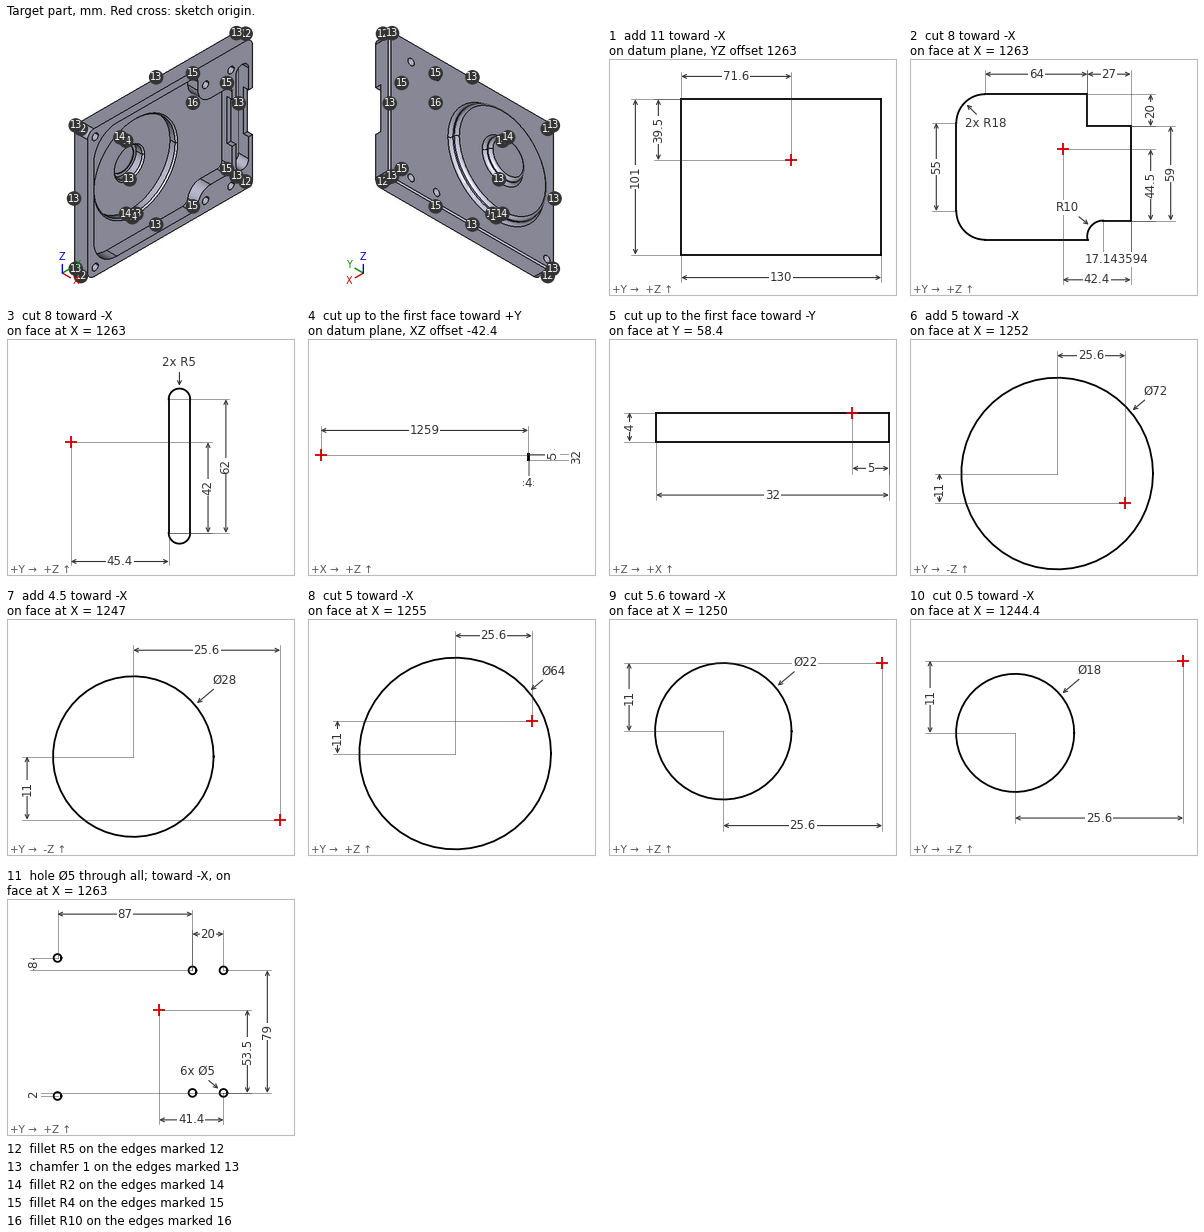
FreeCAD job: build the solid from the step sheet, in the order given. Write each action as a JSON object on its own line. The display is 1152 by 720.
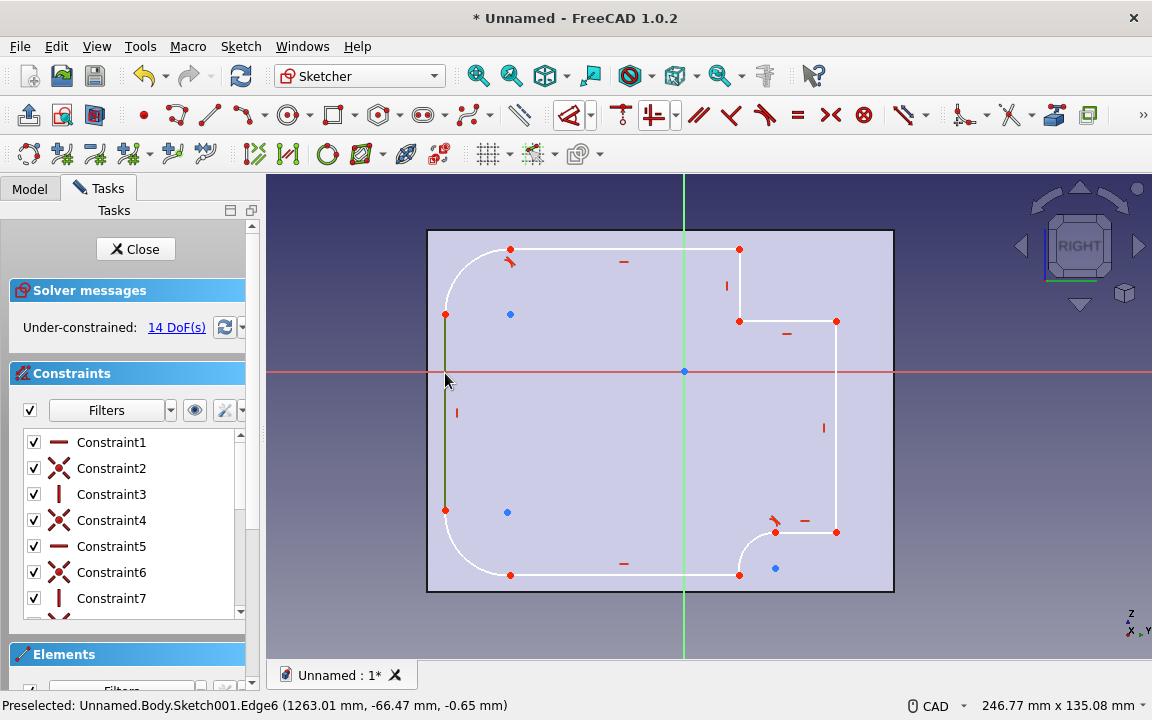
{"action": "left_click", "coordinate": [481, 256]}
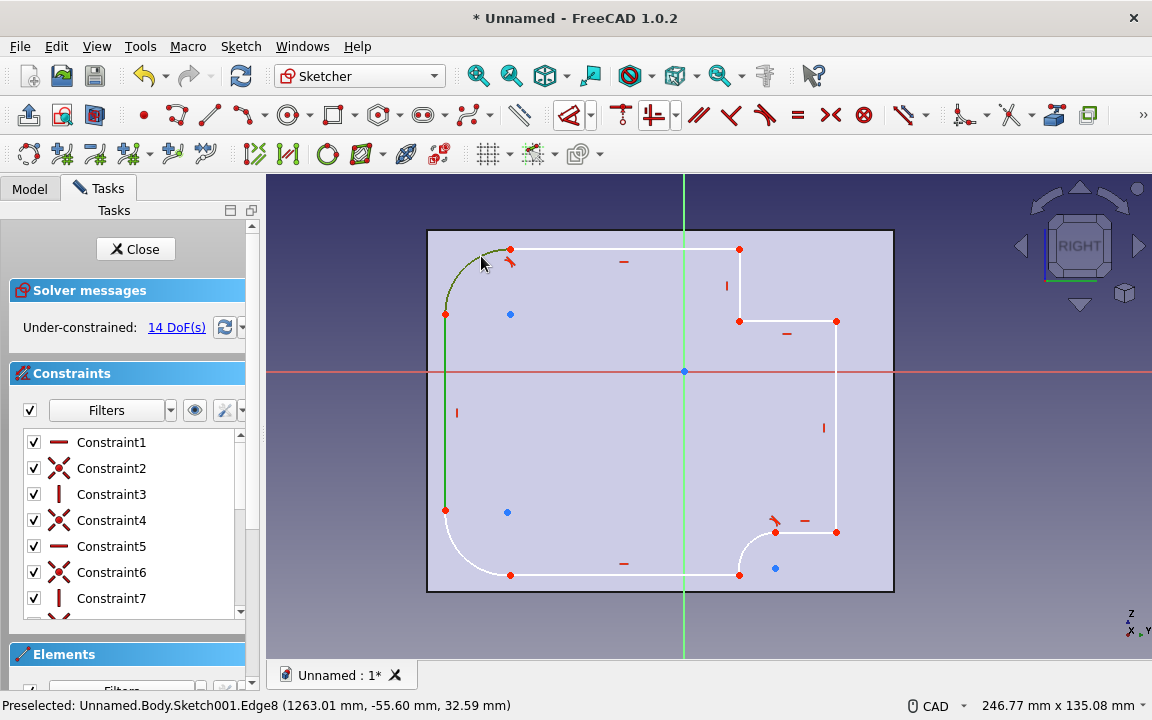
{"action": "left_click", "coordinate": [765, 116]}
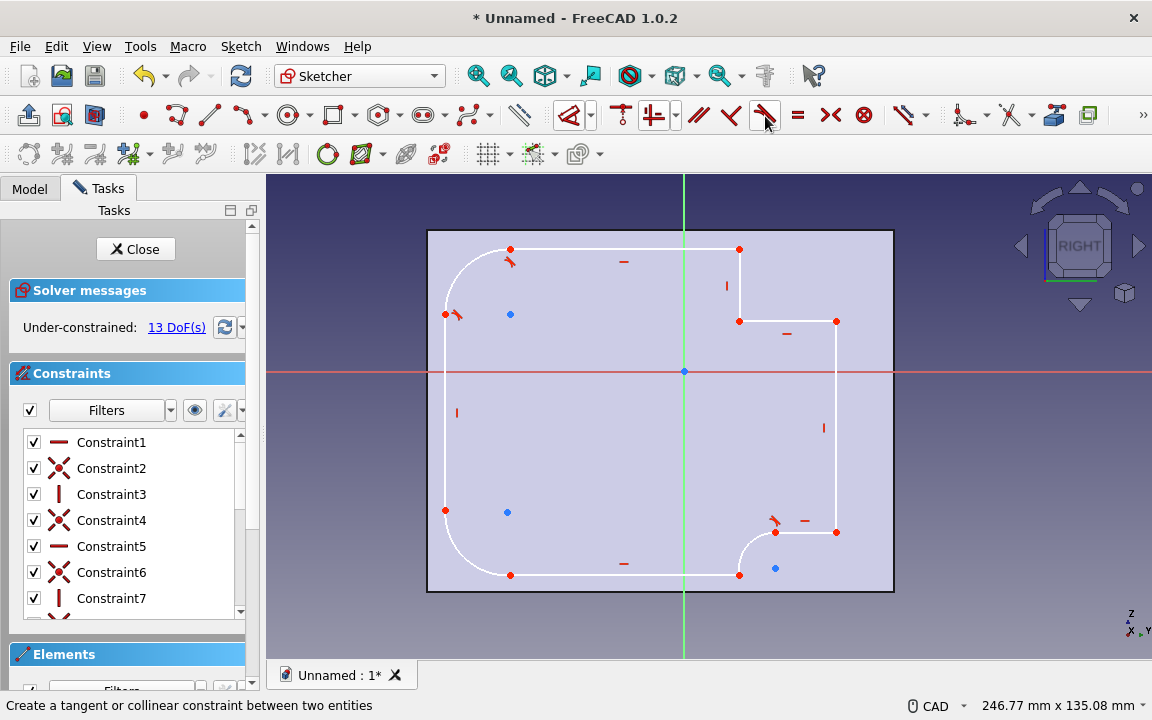
{"action": "left_click", "coordinate": [445, 373]}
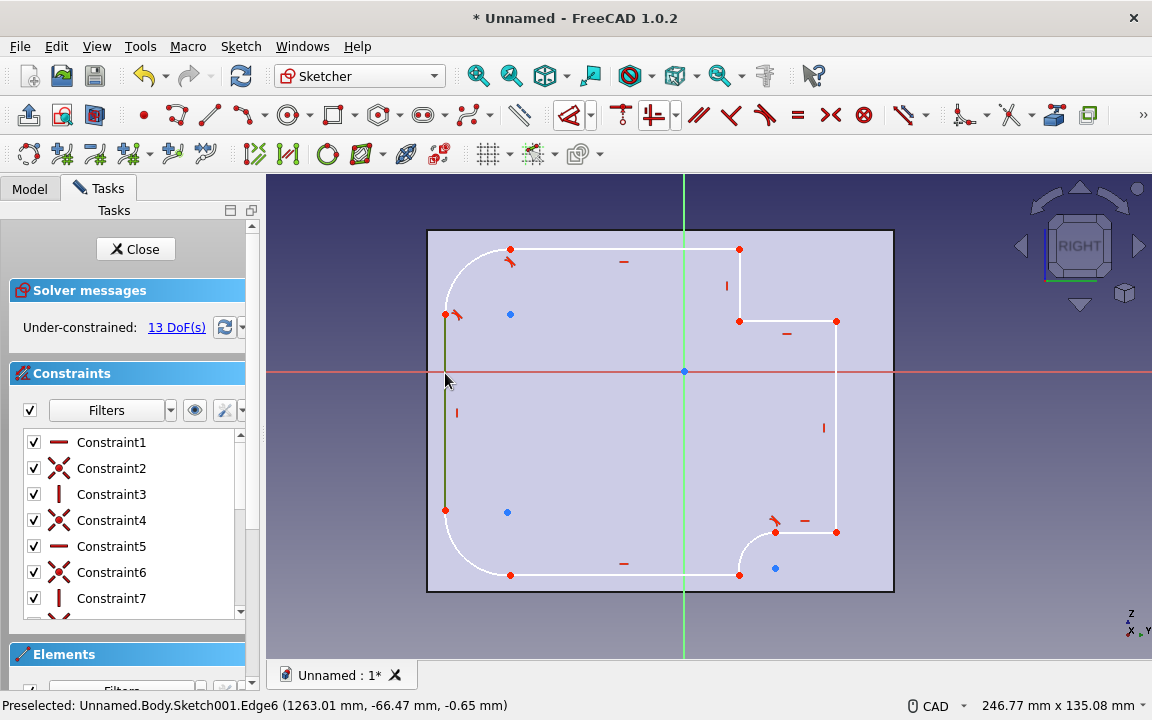
{"action": "left_click", "coordinate": [452, 541]}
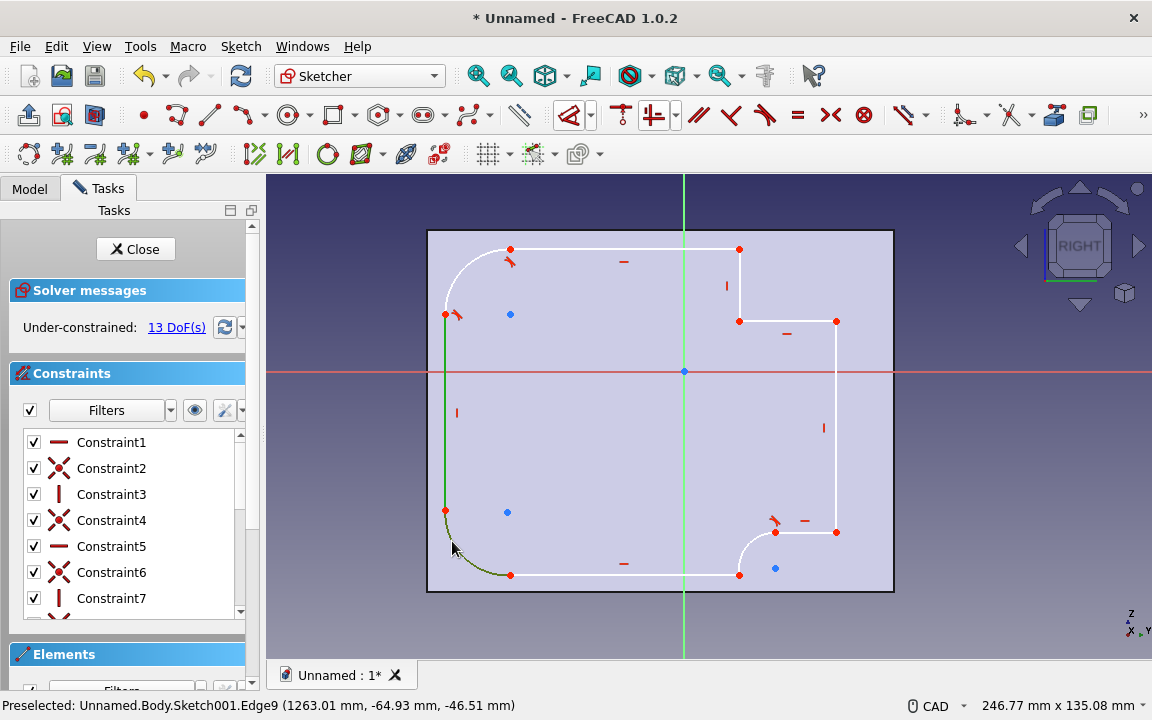
{"action": "left_click", "coordinate": [765, 116]}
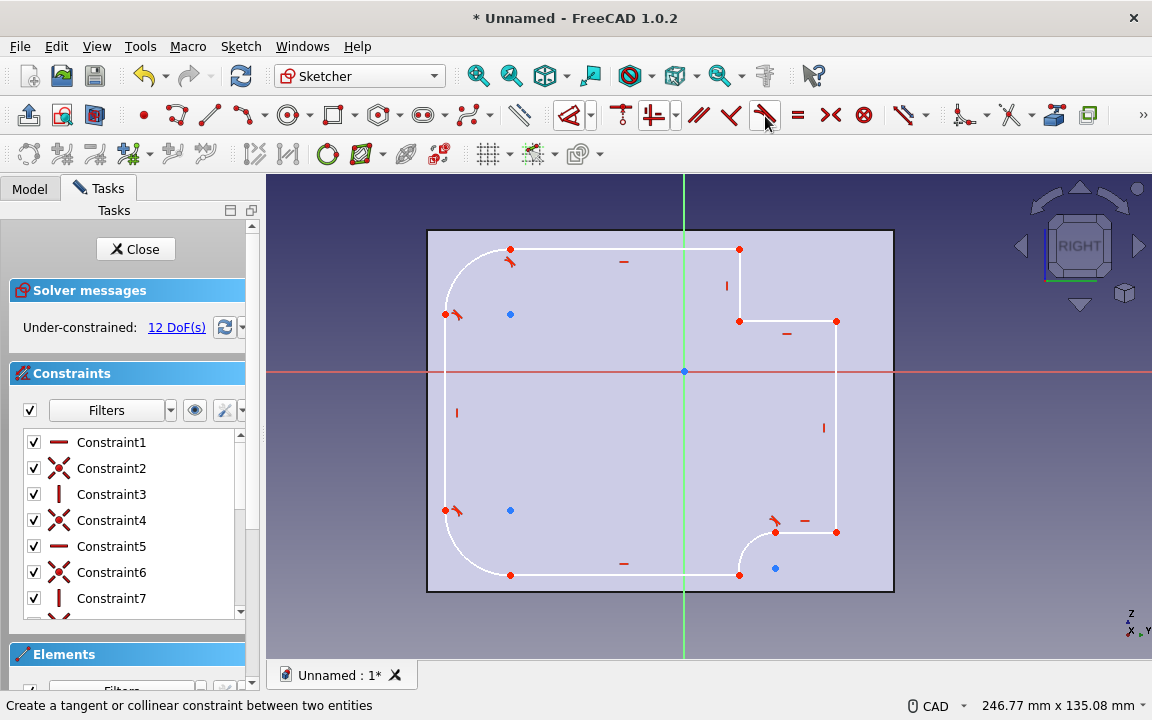
{"action": "left_click", "coordinate": [579, 575]}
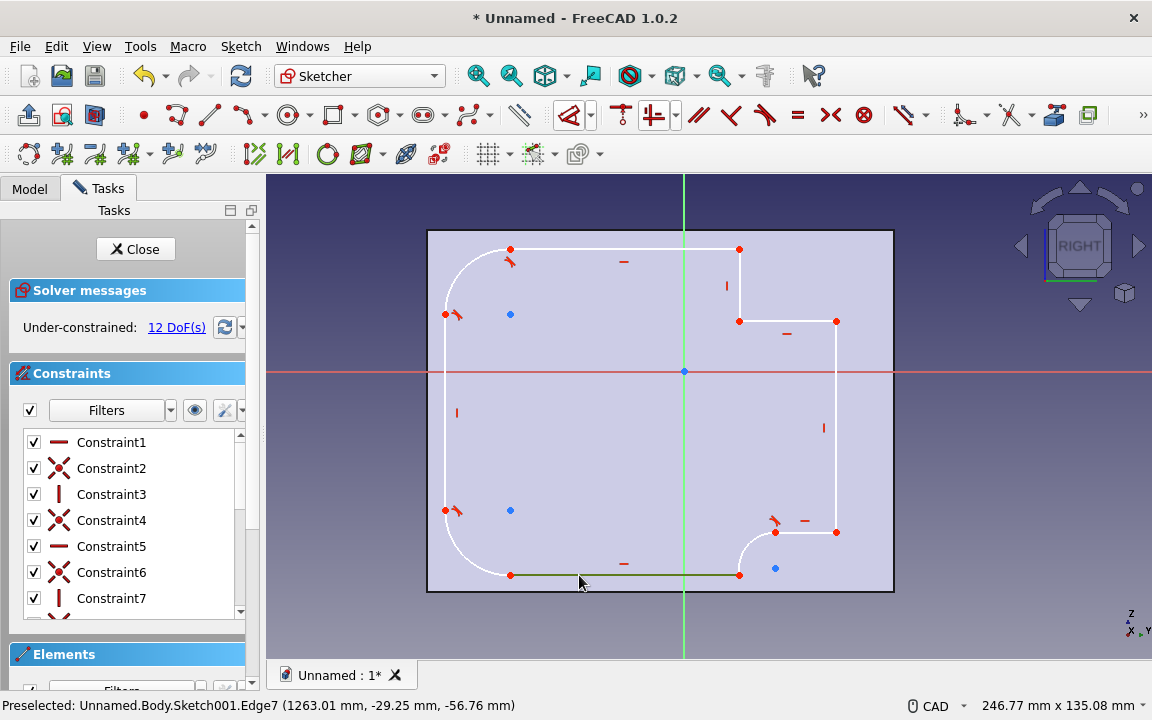
{"action": "left_click", "coordinate": [452, 540]}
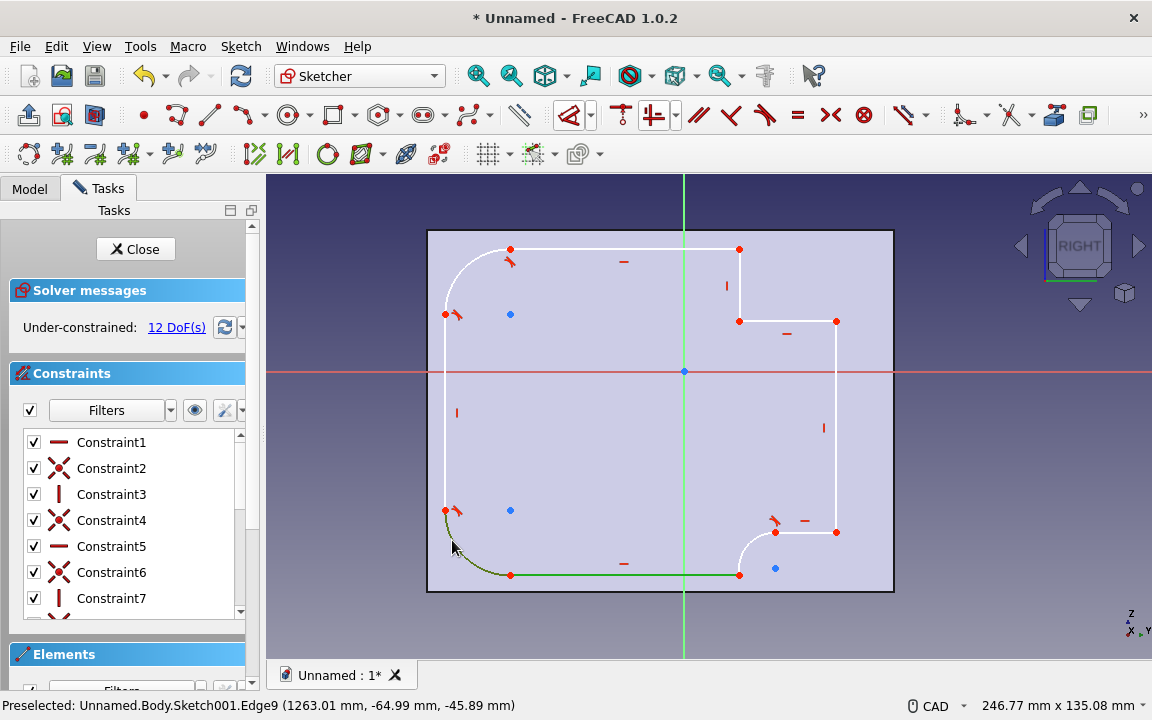
{"action": "left_click", "coordinate": [765, 116]}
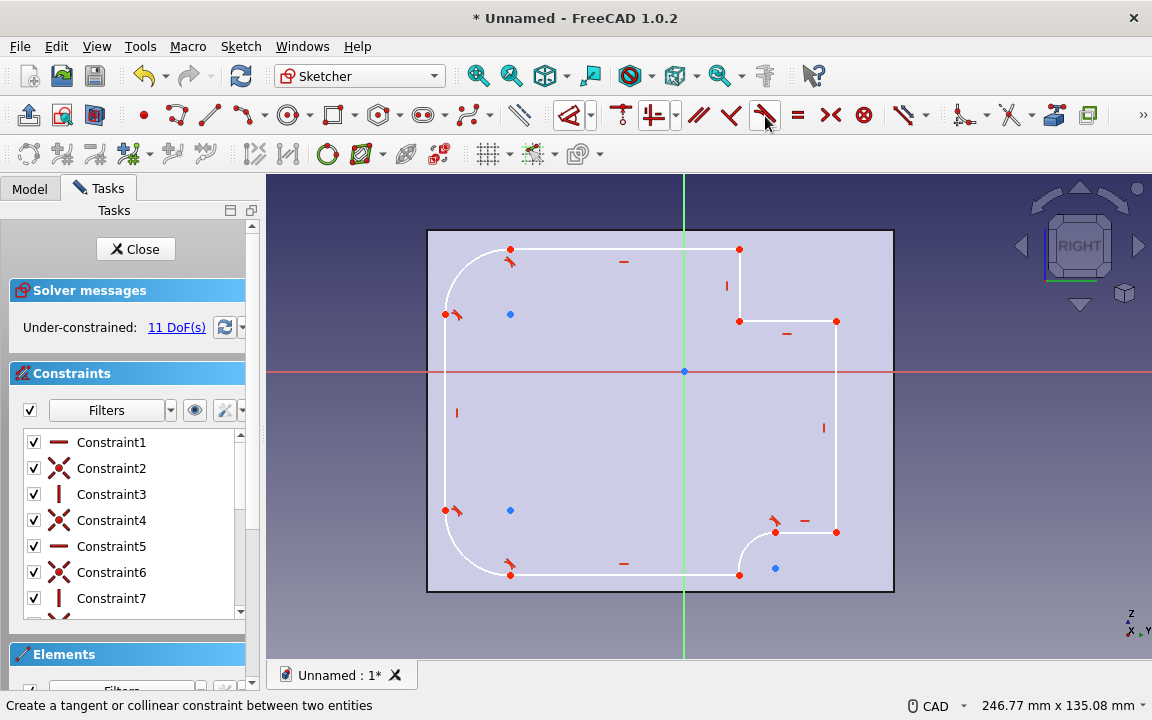
{"action": "left_click", "coordinate": [481, 256]}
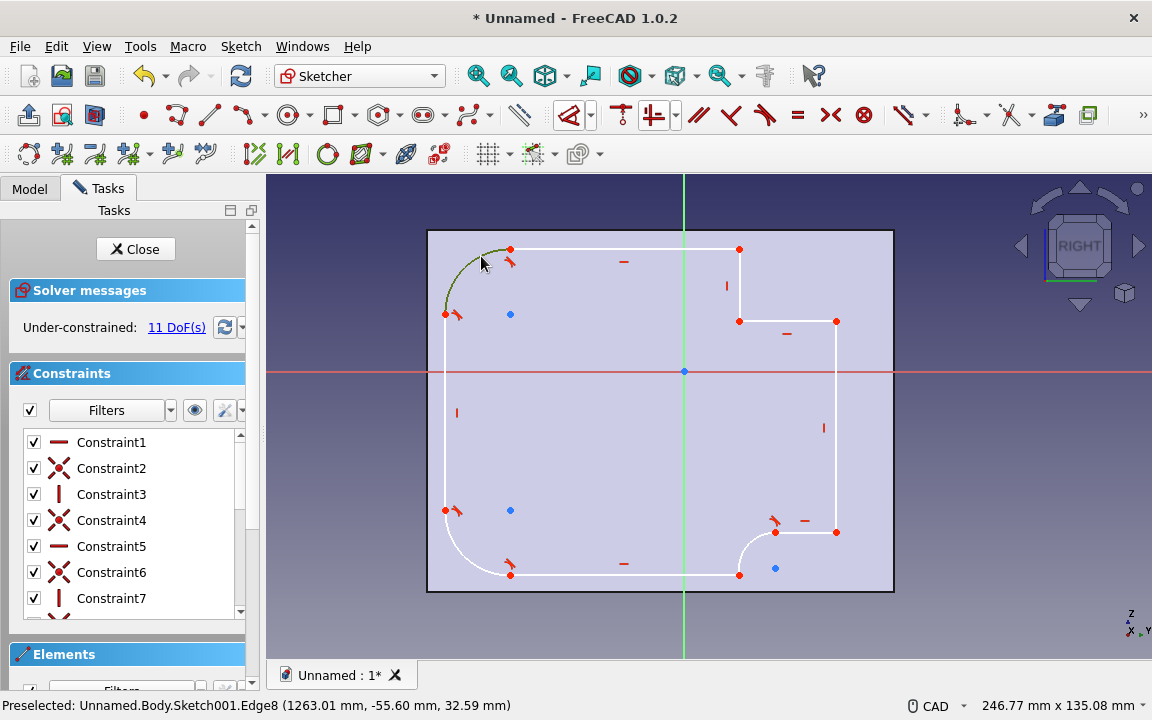
{"action": "left_click", "coordinate": [452, 540]}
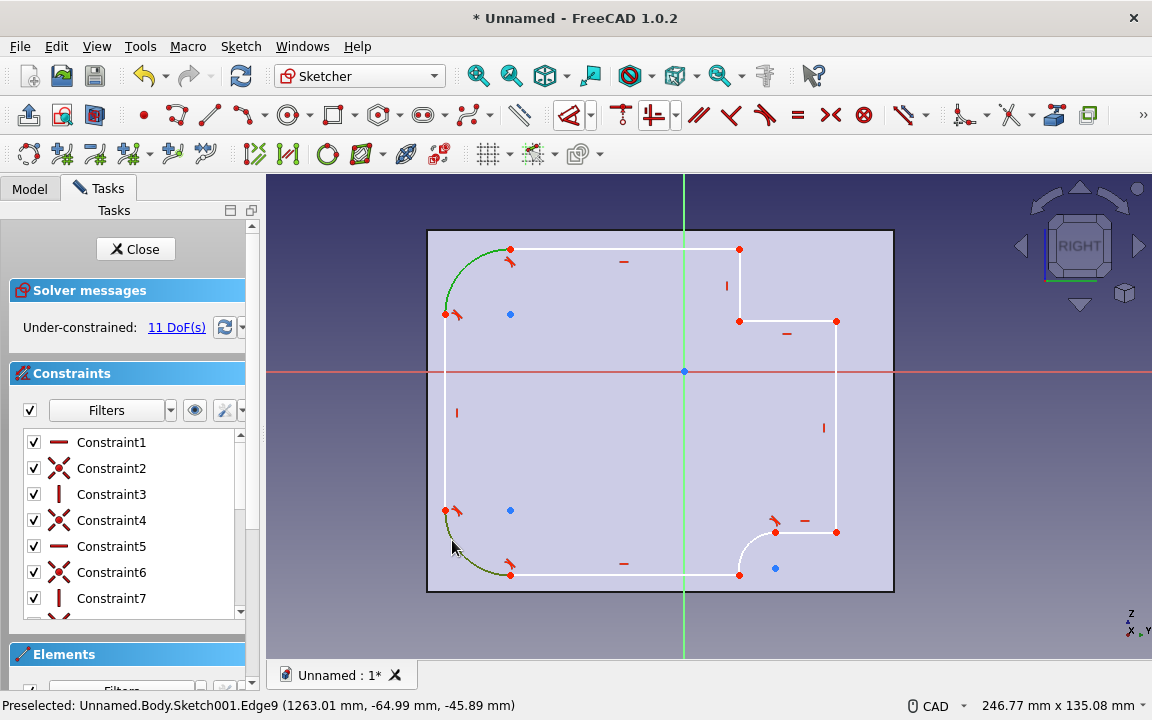
{"action": "left_click", "coordinate": [798, 116]}